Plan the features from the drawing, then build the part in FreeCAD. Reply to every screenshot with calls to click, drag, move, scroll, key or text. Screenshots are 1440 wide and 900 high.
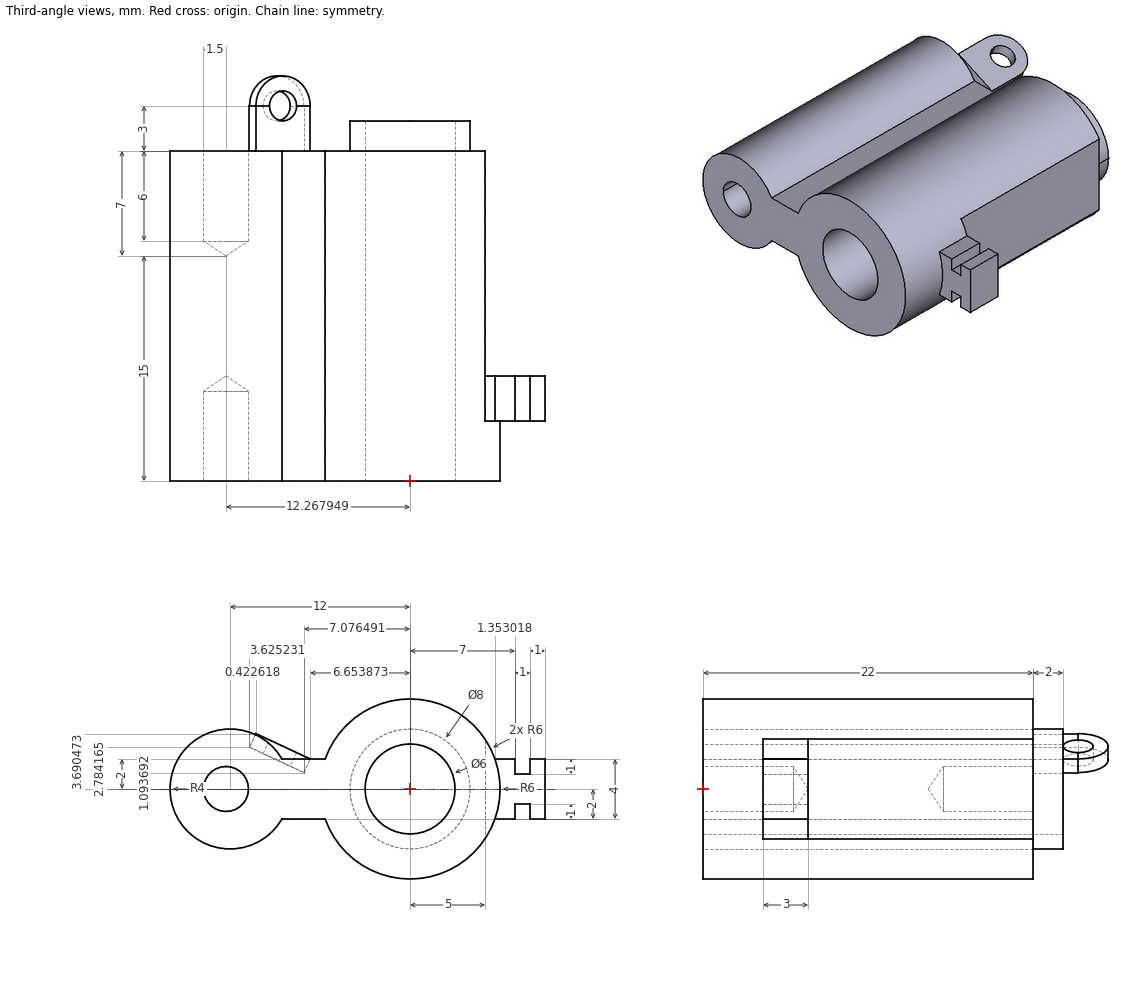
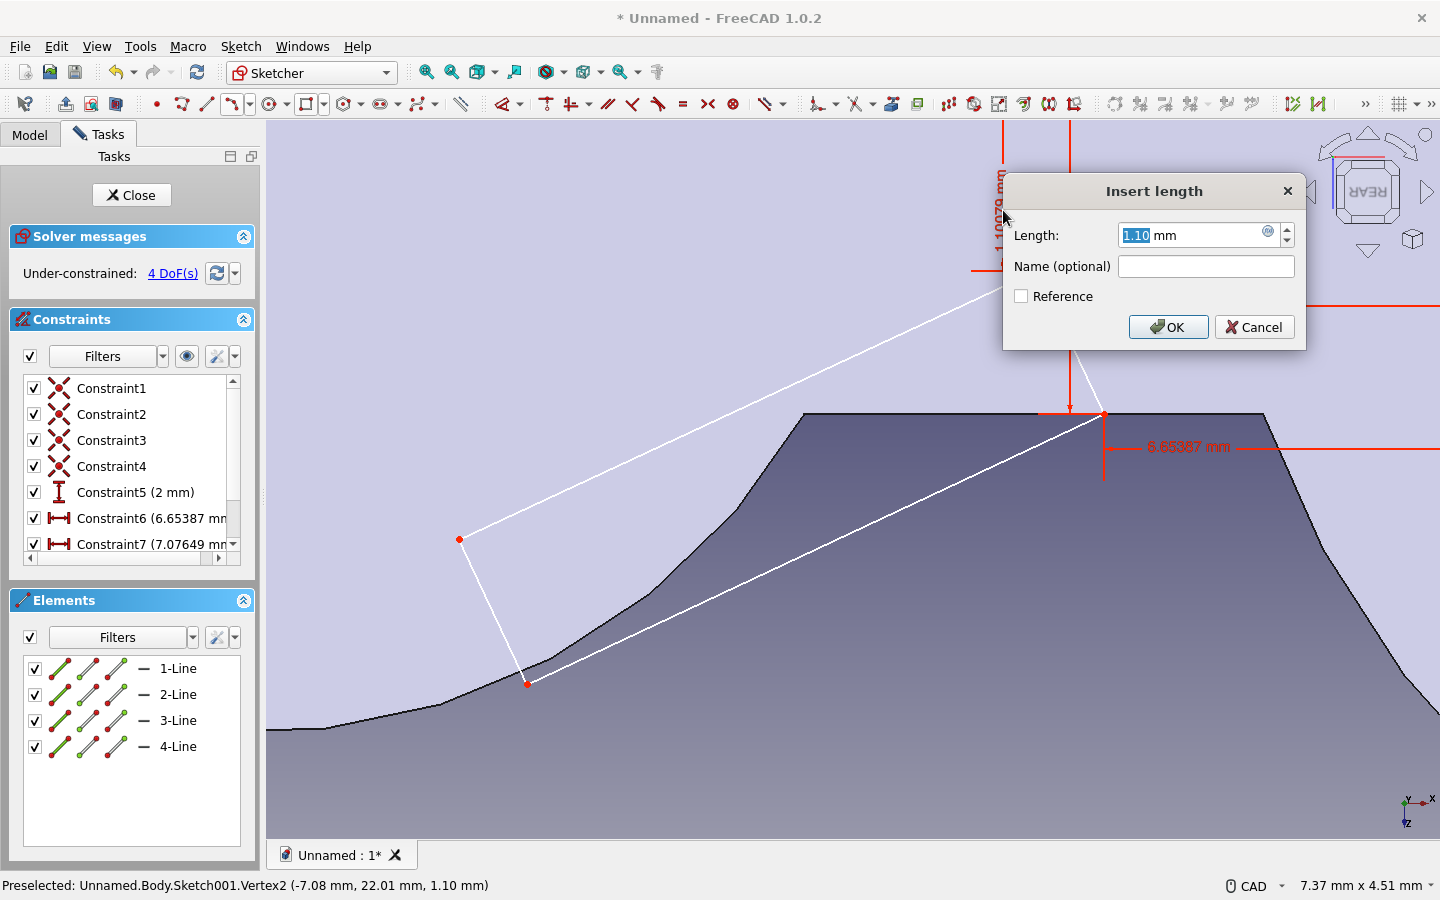
text(1.093692)
key(Return)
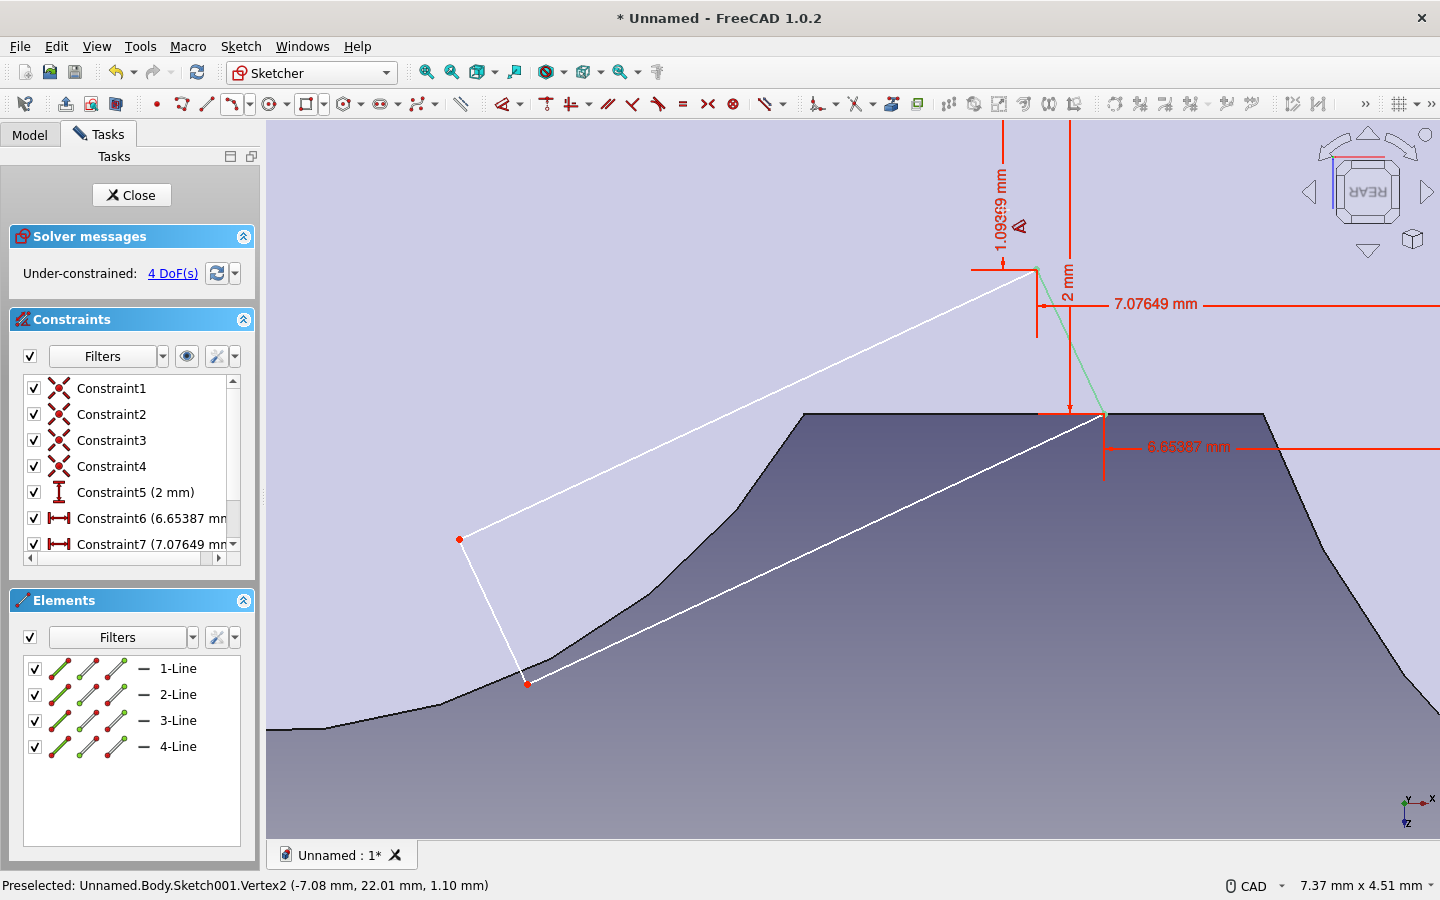
click(459, 540)
click(425, 344)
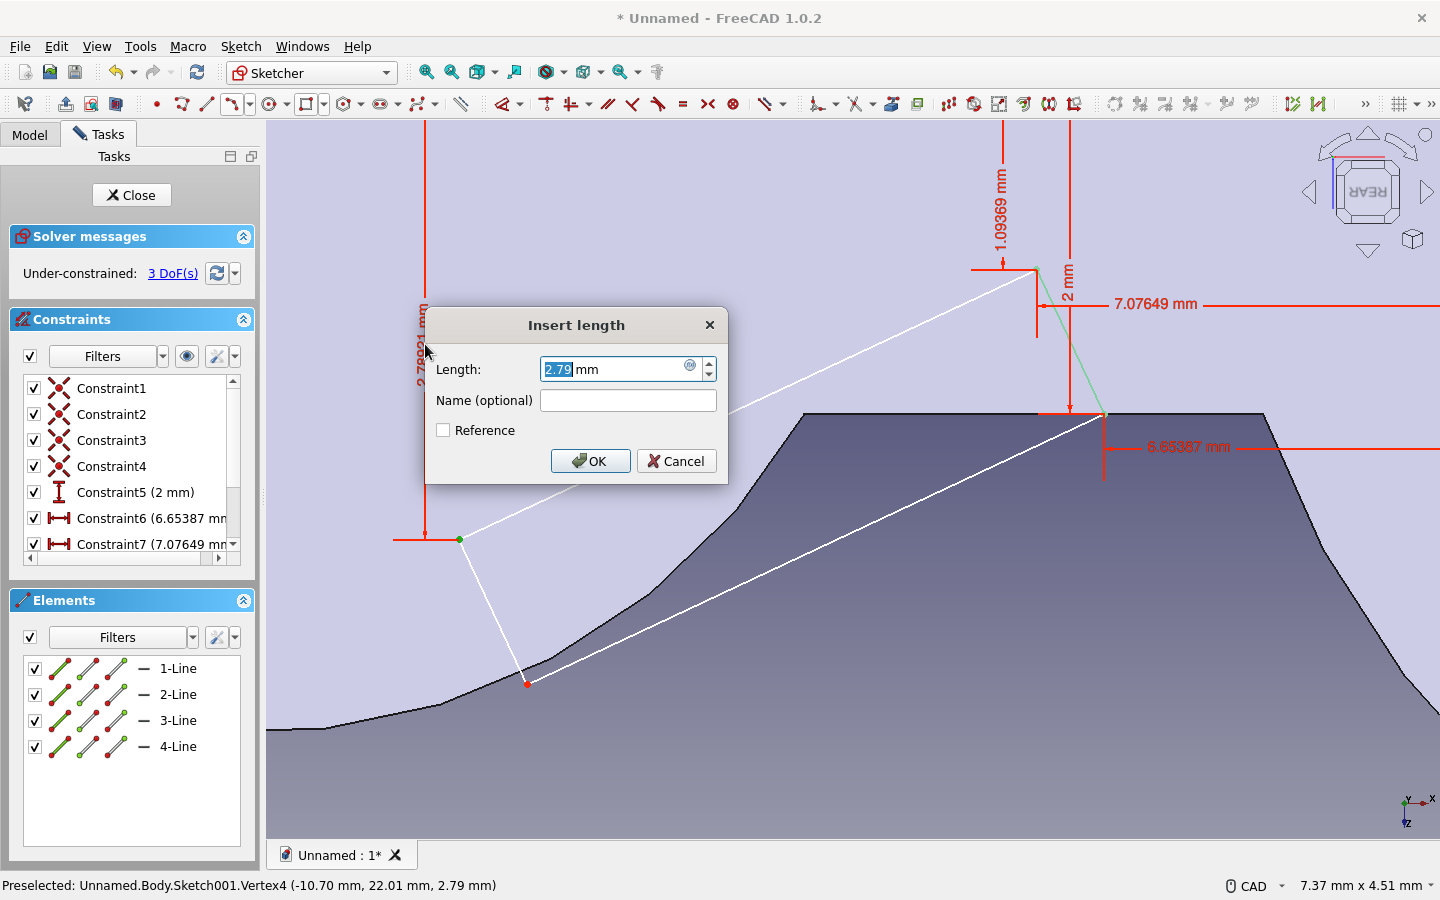
text(2.784165)
key(Return)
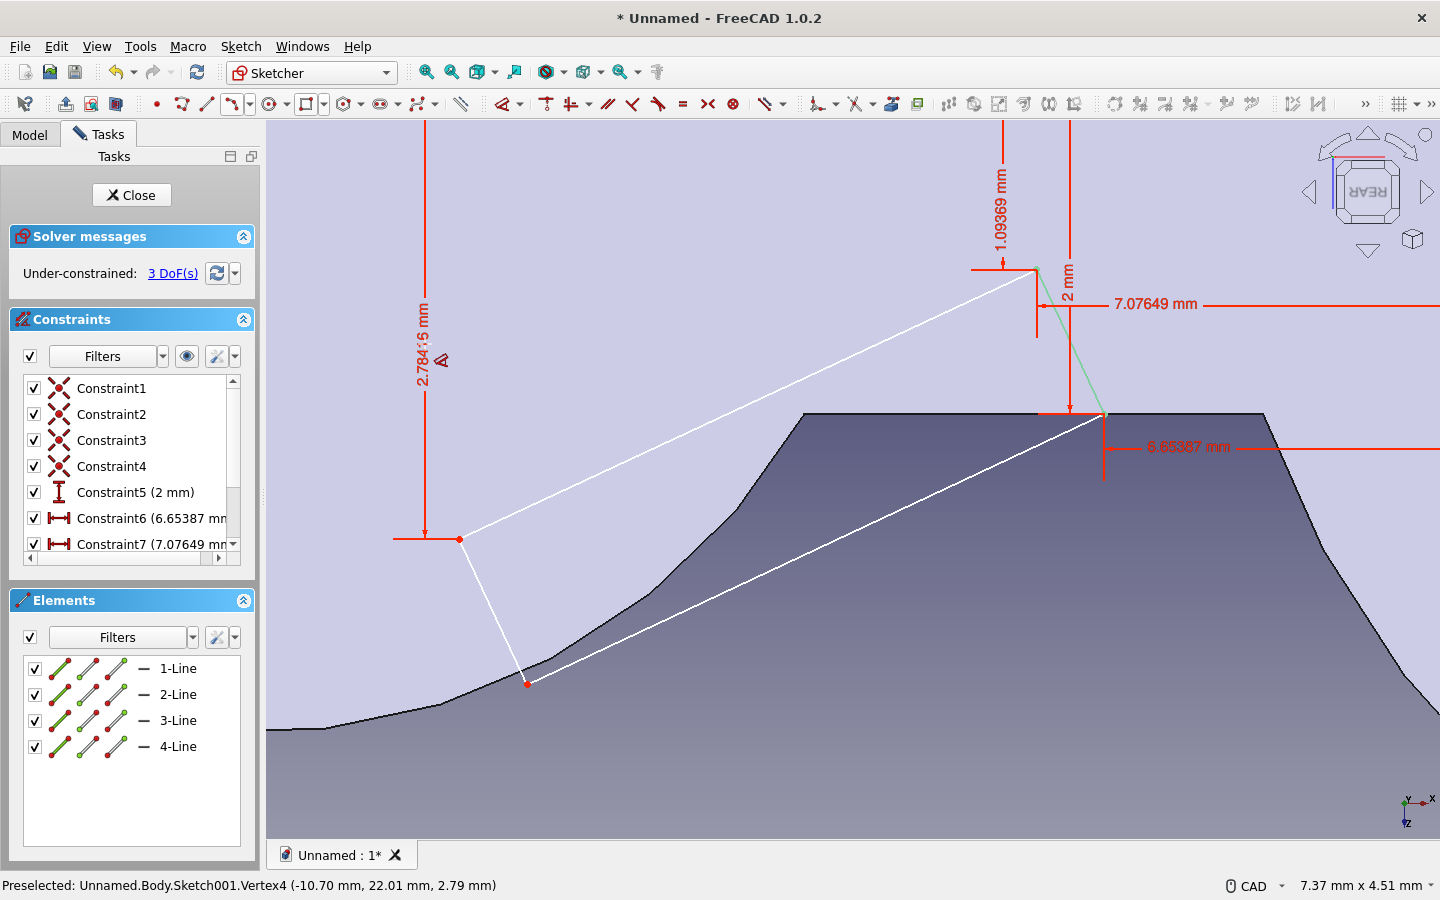
click(527, 685)
click(493, 416)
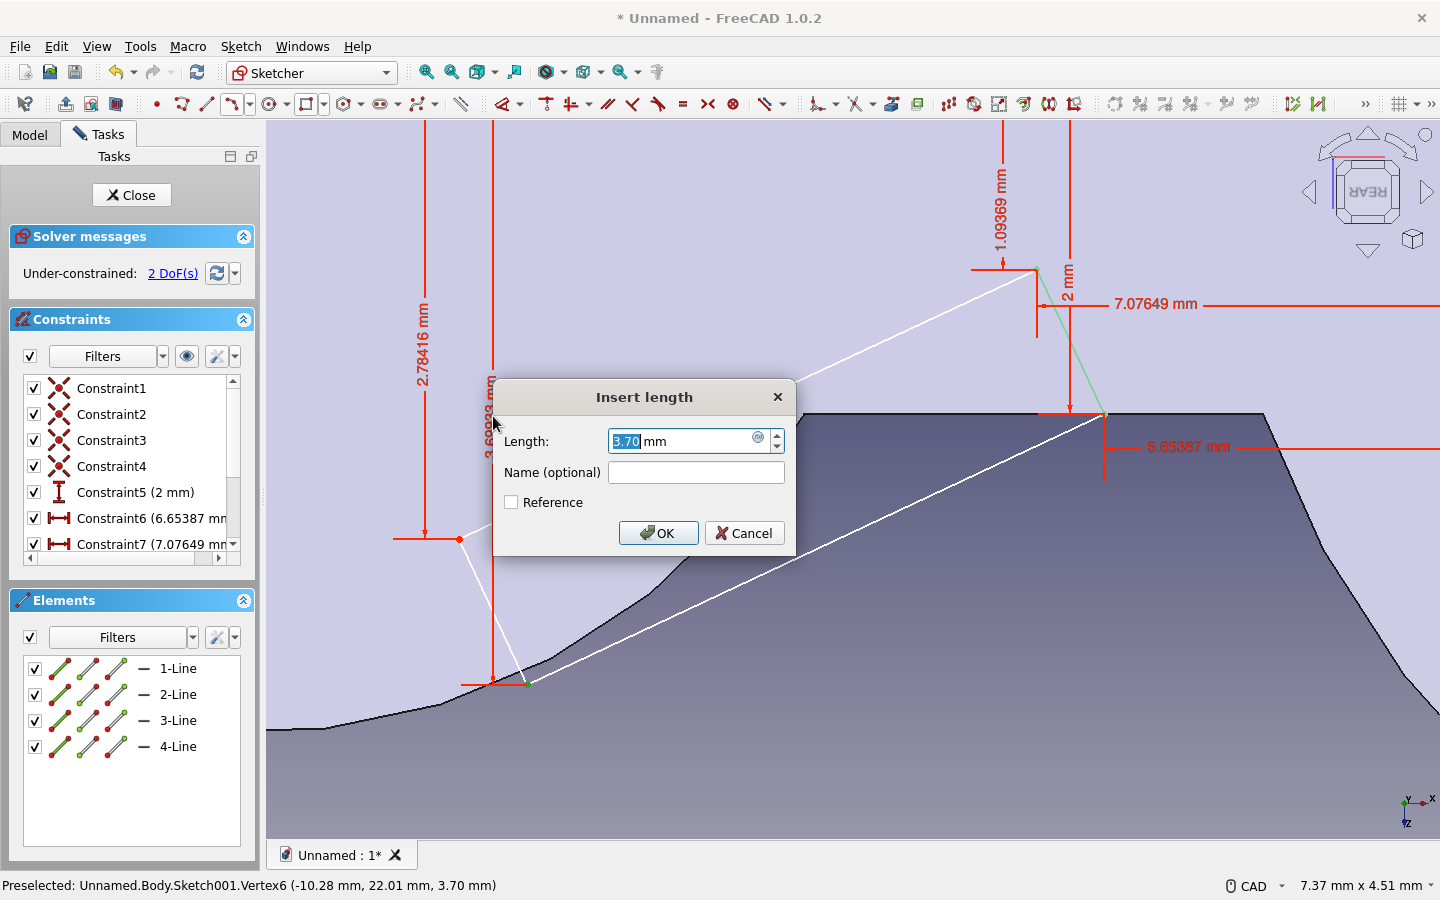
text(3.690473)
key(Return)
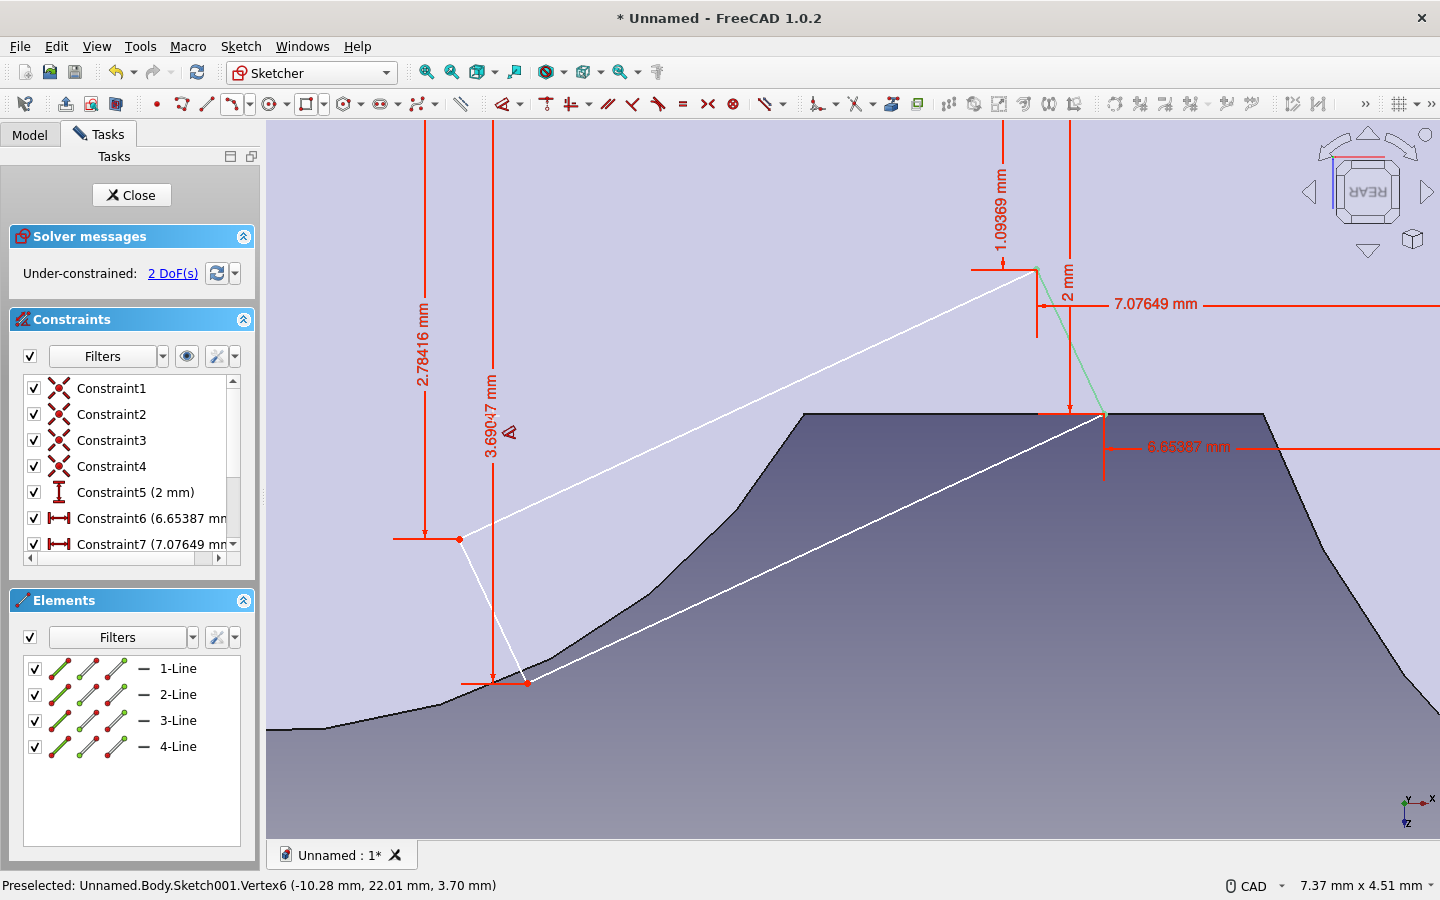
click(864, 351)
click(748, 236)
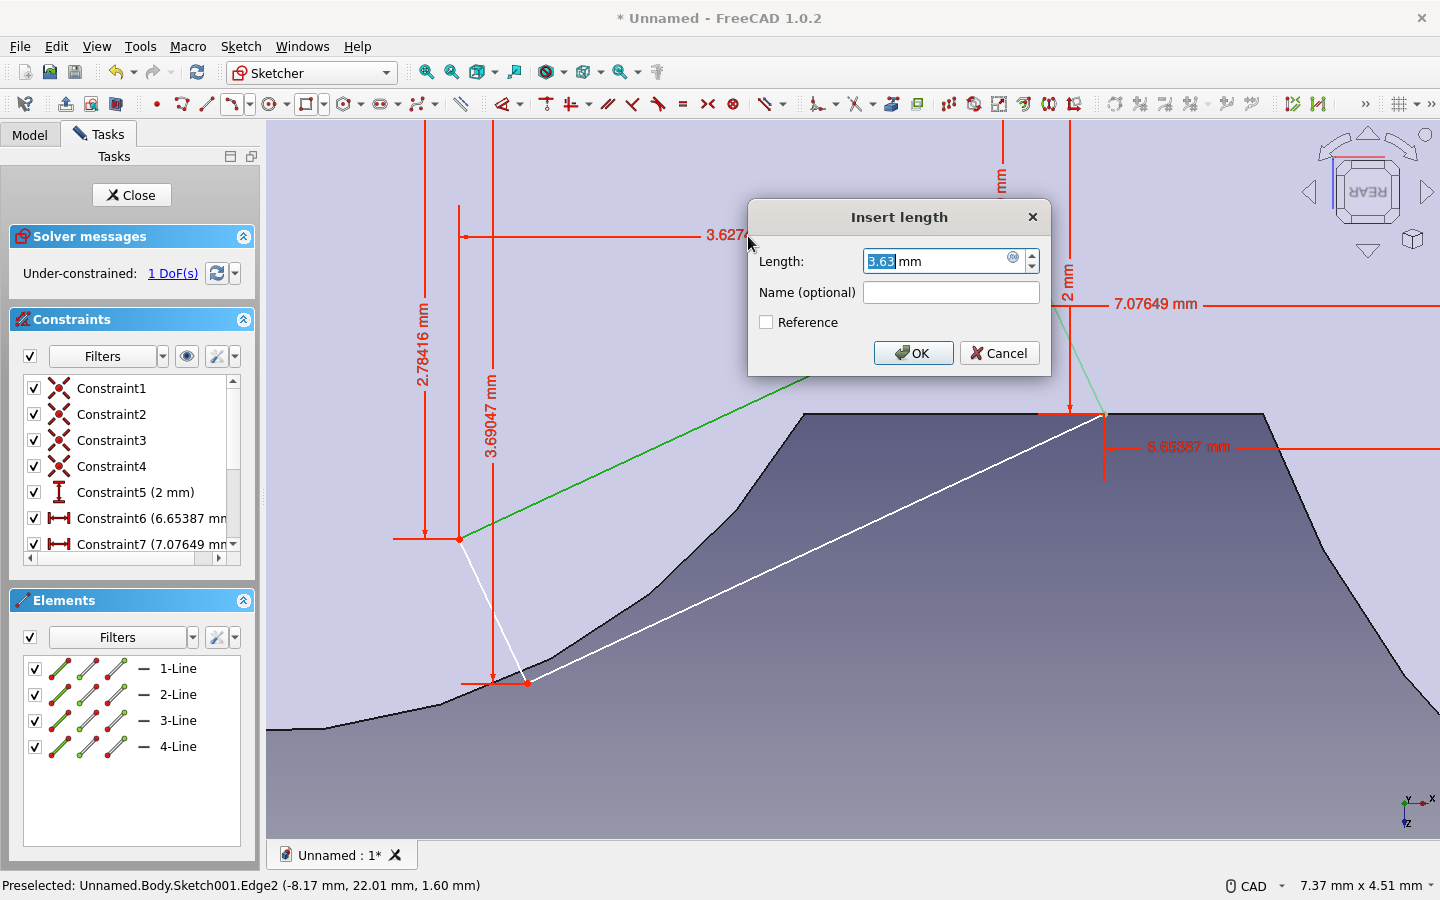
text(3.625231)
key(Return)